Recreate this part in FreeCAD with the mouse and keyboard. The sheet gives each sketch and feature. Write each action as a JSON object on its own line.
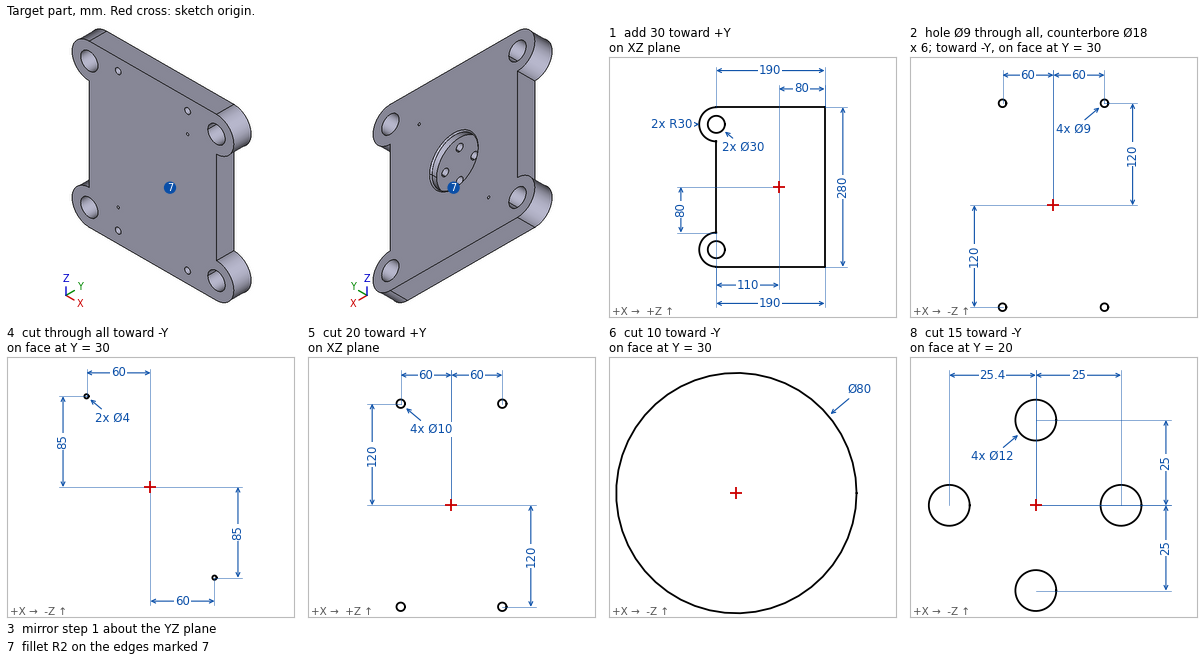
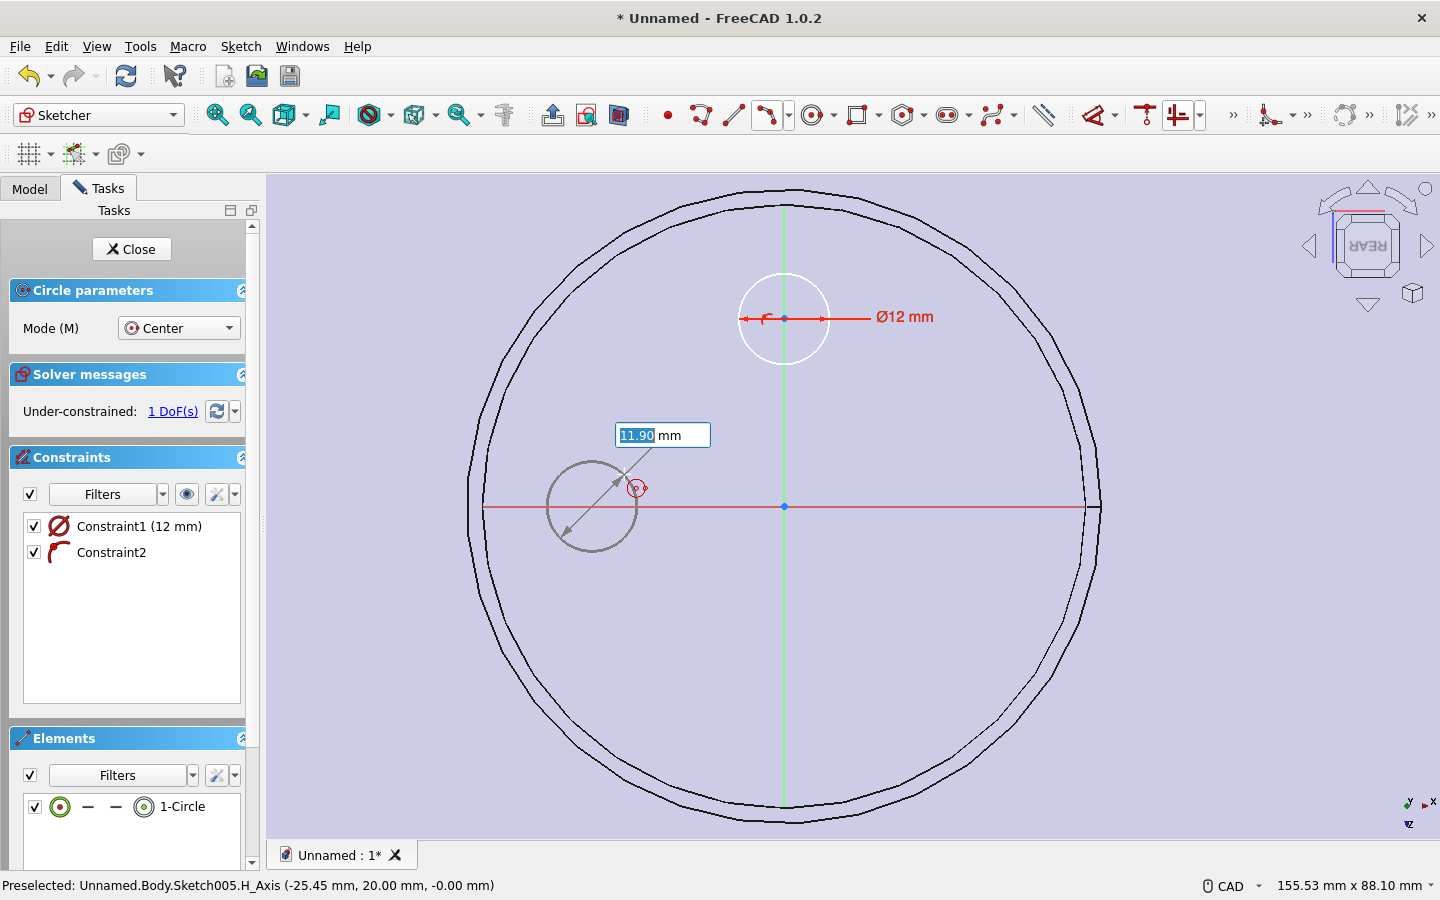
{"action": "type", "text": "12"}
{"action": "key", "text": "Return"}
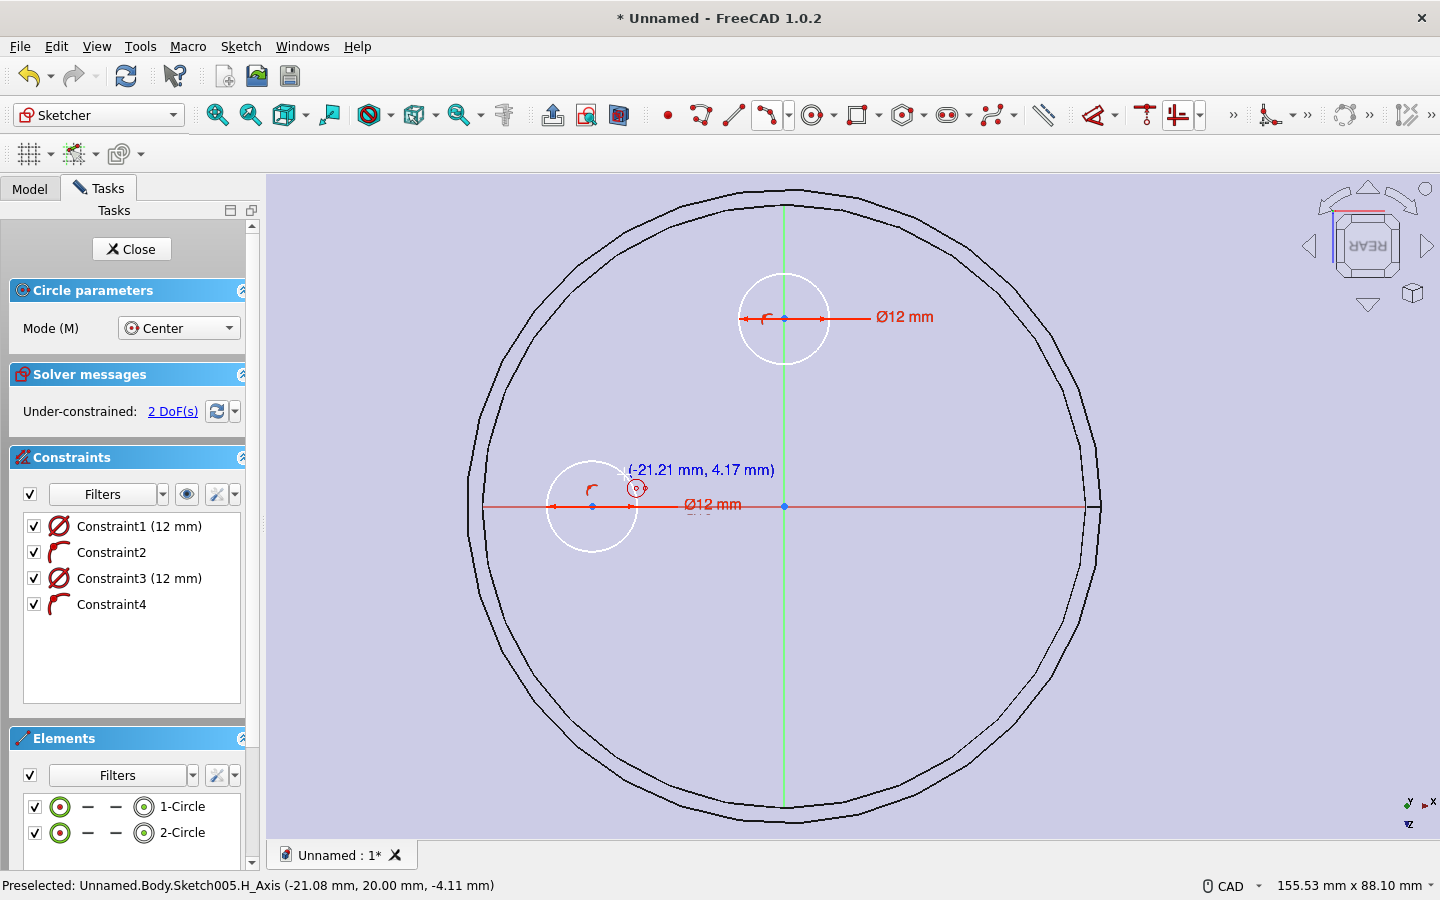
{"action": "left_click", "coordinate": [973, 506]}
{"action": "mouse_move", "coordinate": [1005, 474]}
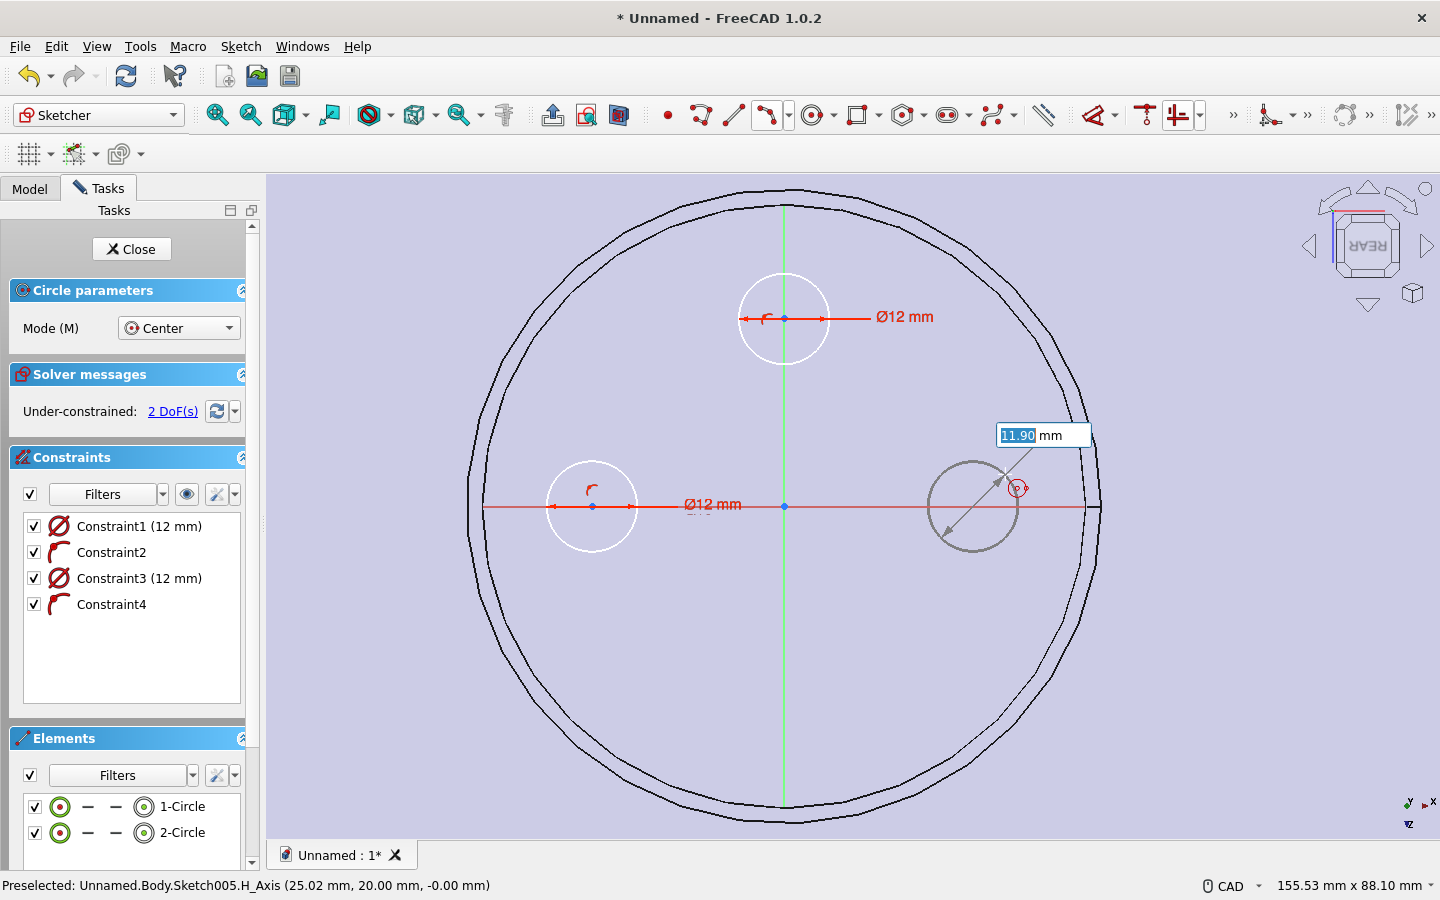
{"action": "type", "text": "12"}
{"action": "key", "text": "Return"}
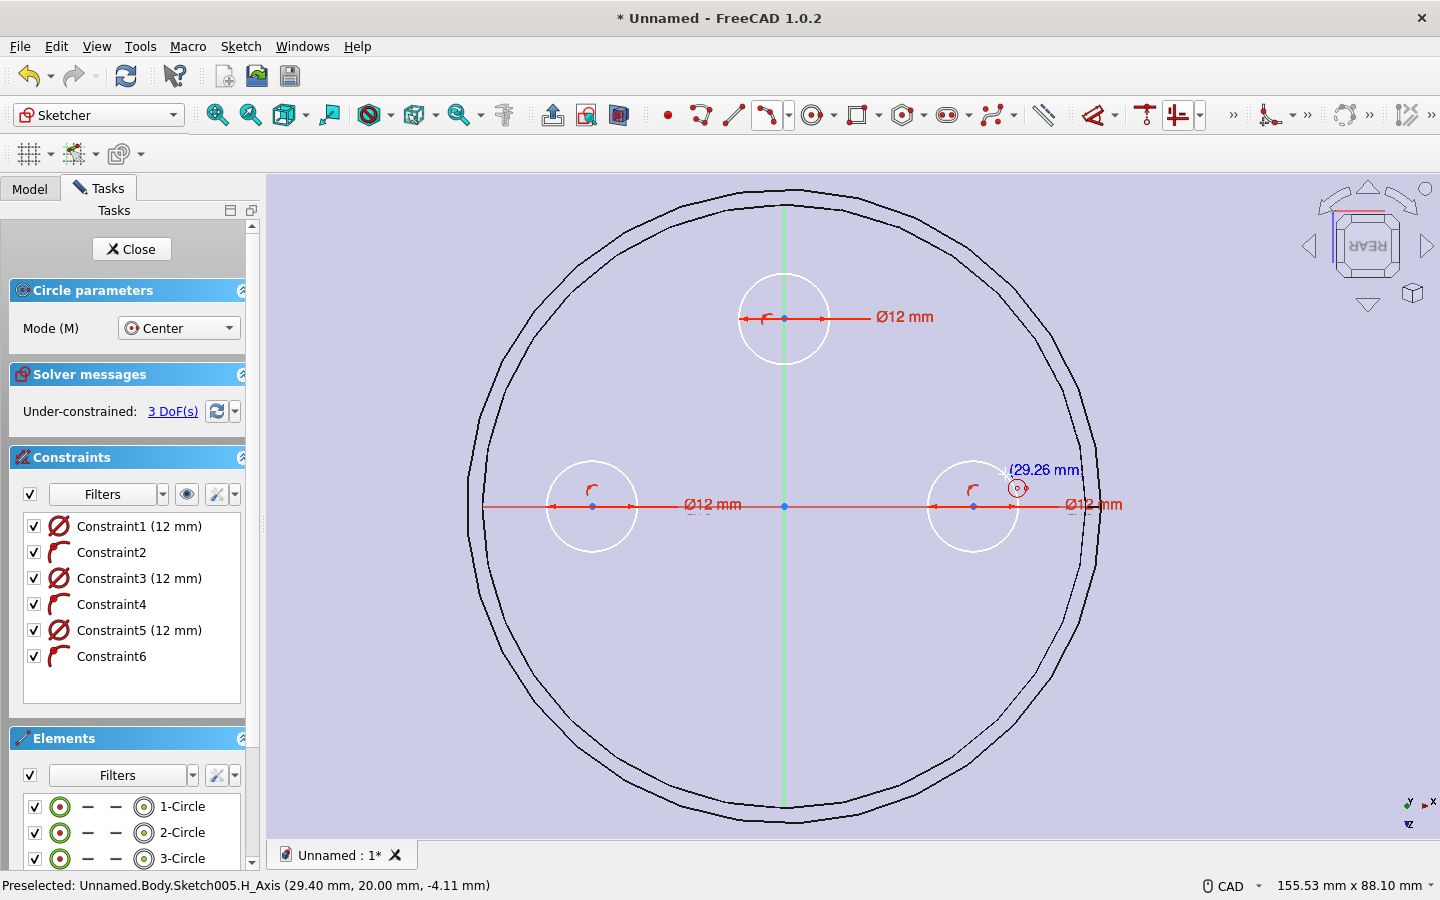
{"action": "left_click", "coordinate": [784, 695]}
{"action": "mouse_move", "coordinate": [816, 663]}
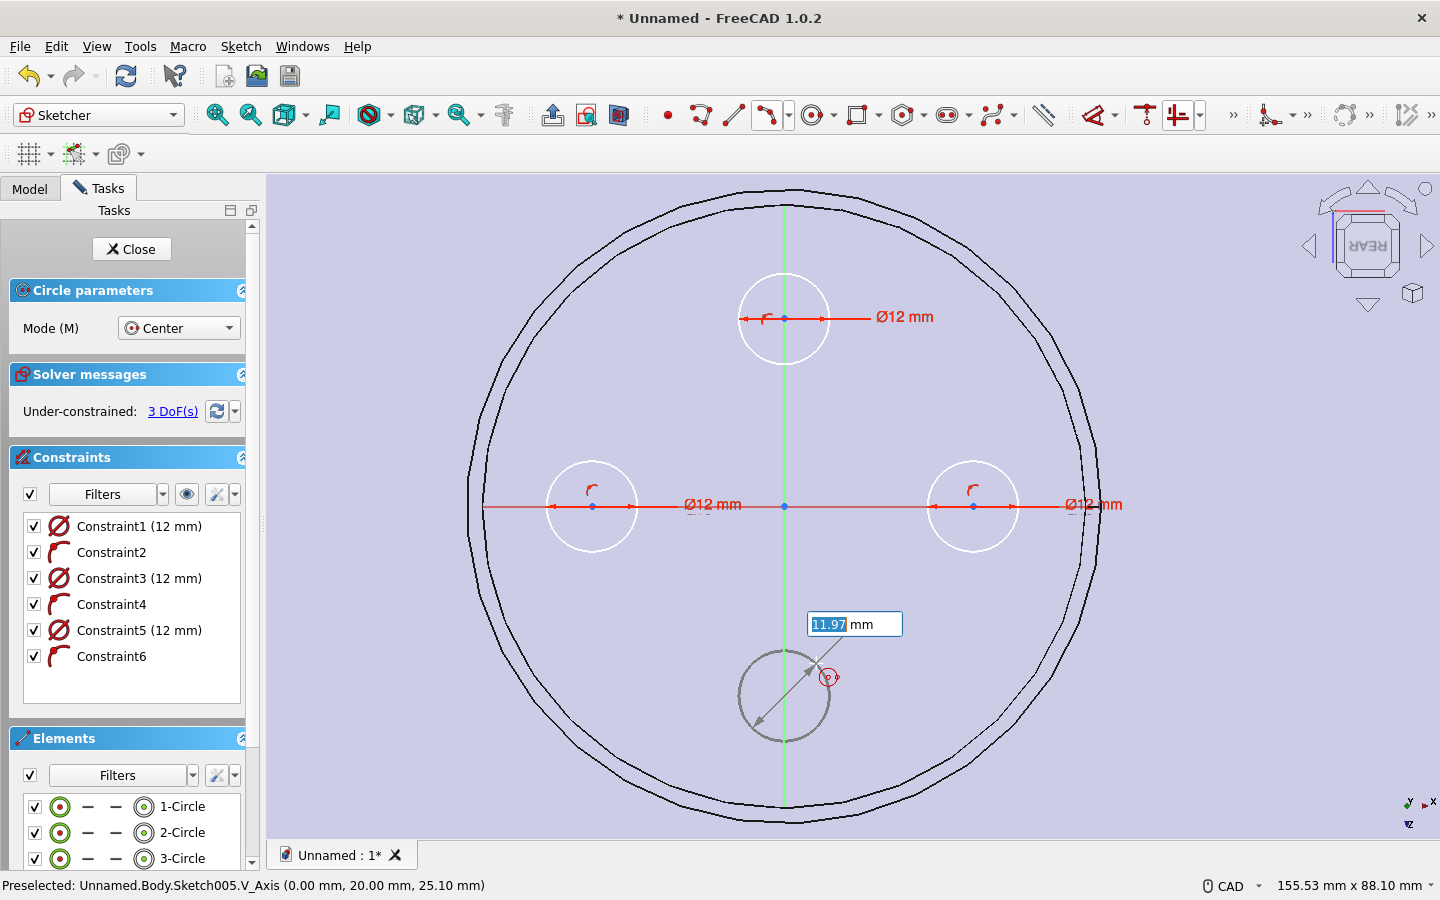
{"action": "type", "text": "12"}
{"action": "key", "text": "Return"}
{"action": "key", "text": "Escape"}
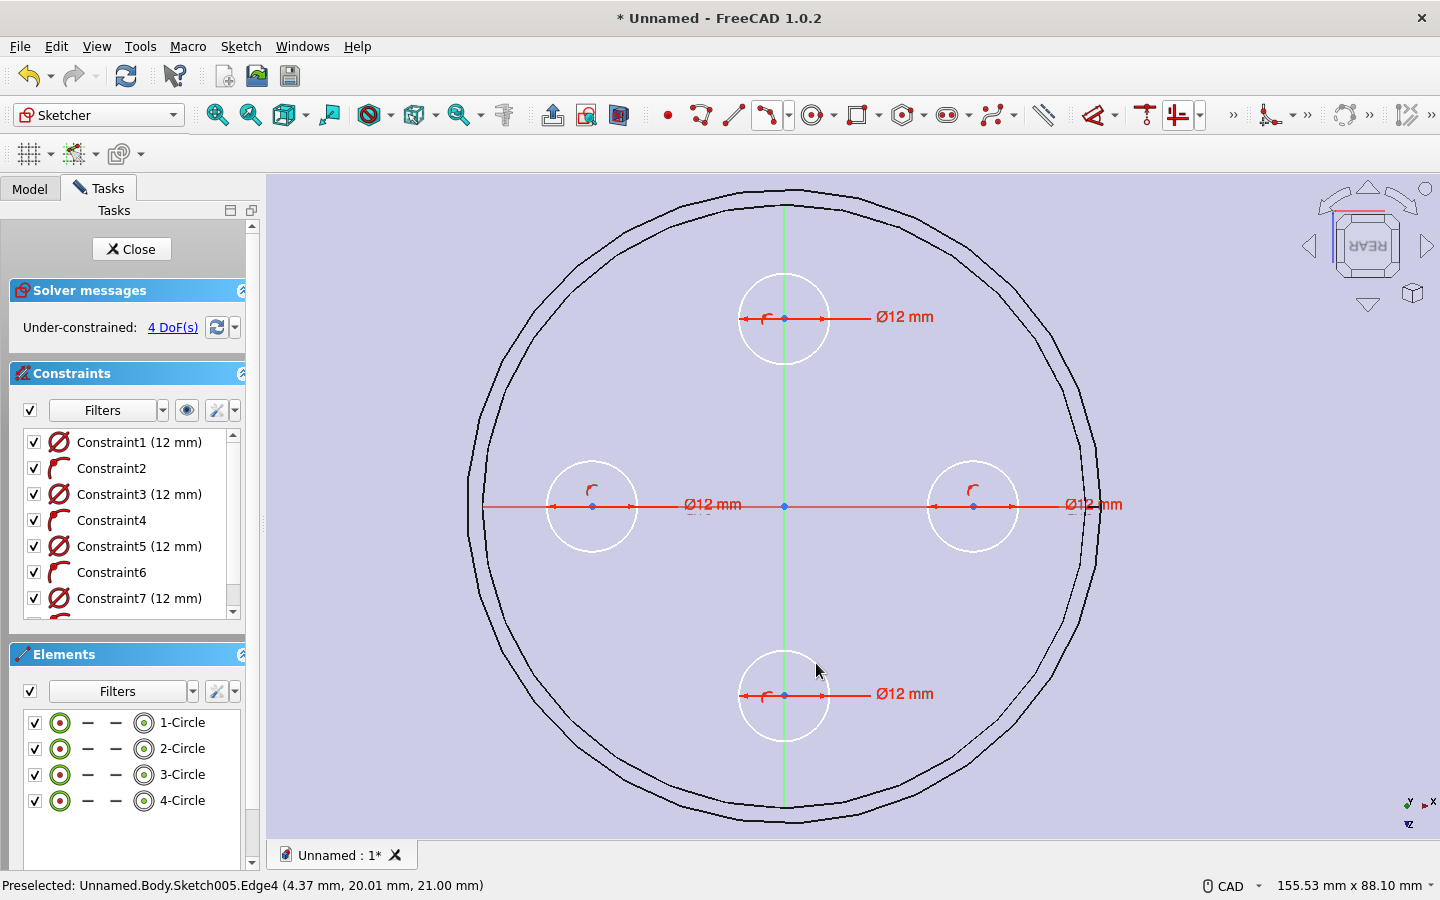
{"action": "left_click", "coordinate": [1092, 116]}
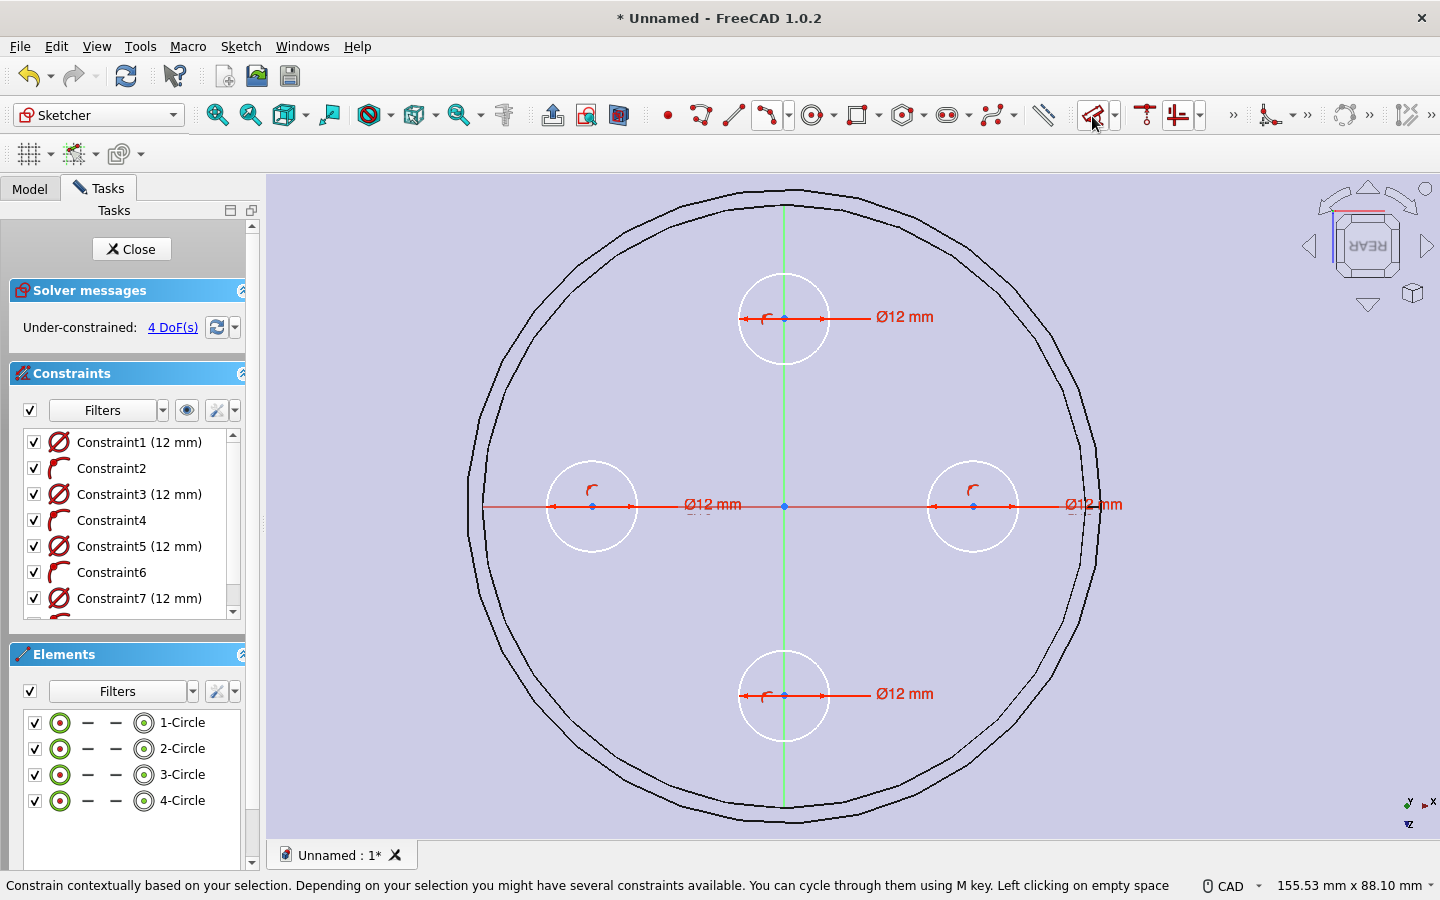
{"action": "left_click", "coordinate": [784, 319]}
{"action": "left_click", "coordinate": [818, 413]}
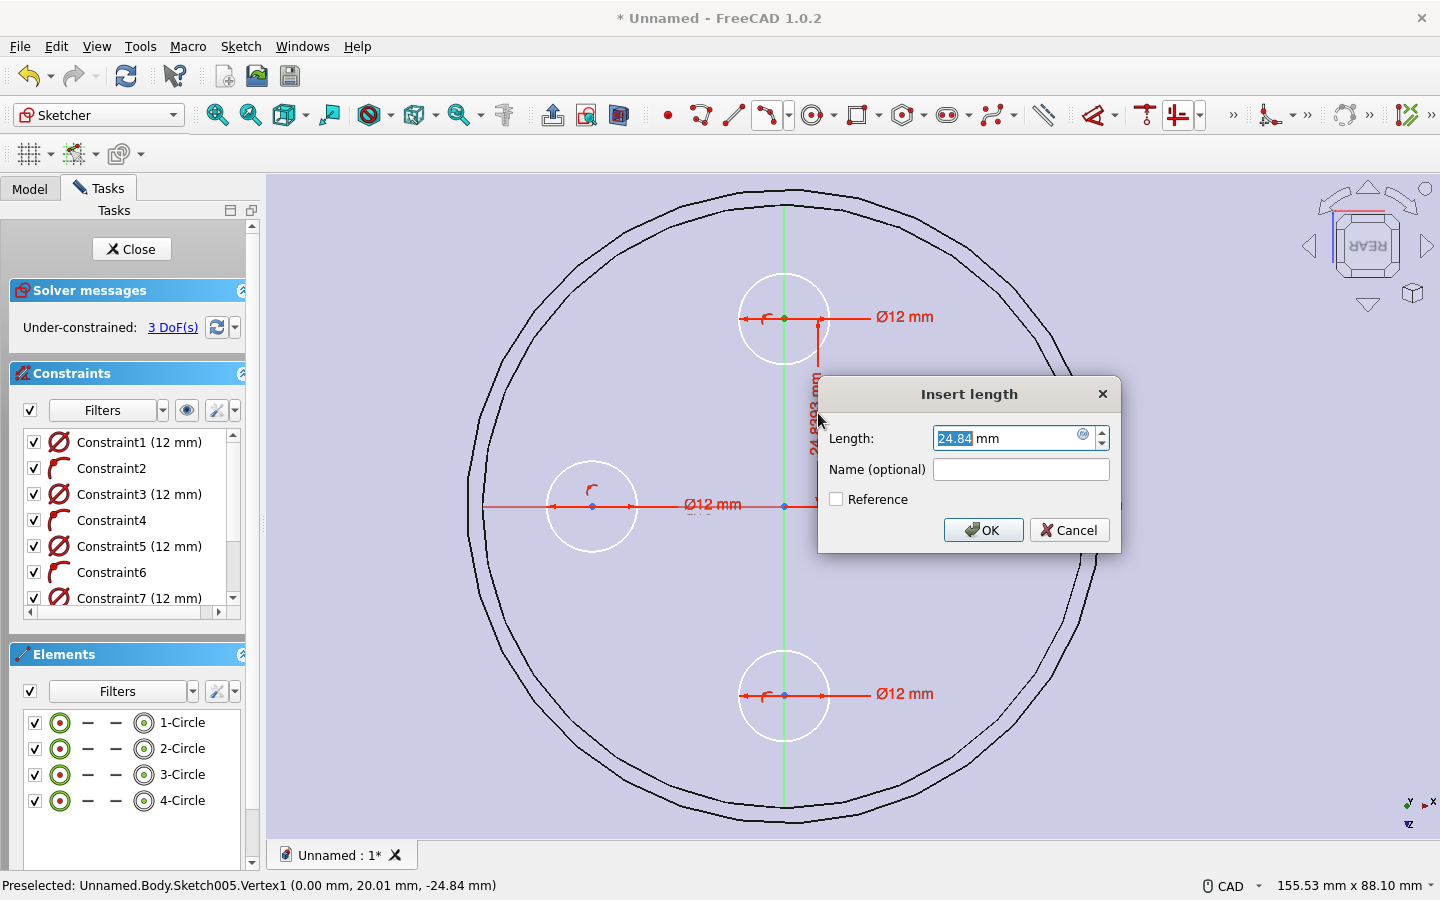
{"action": "type", "text": "25"}
{"action": "key", "text": "Return"}